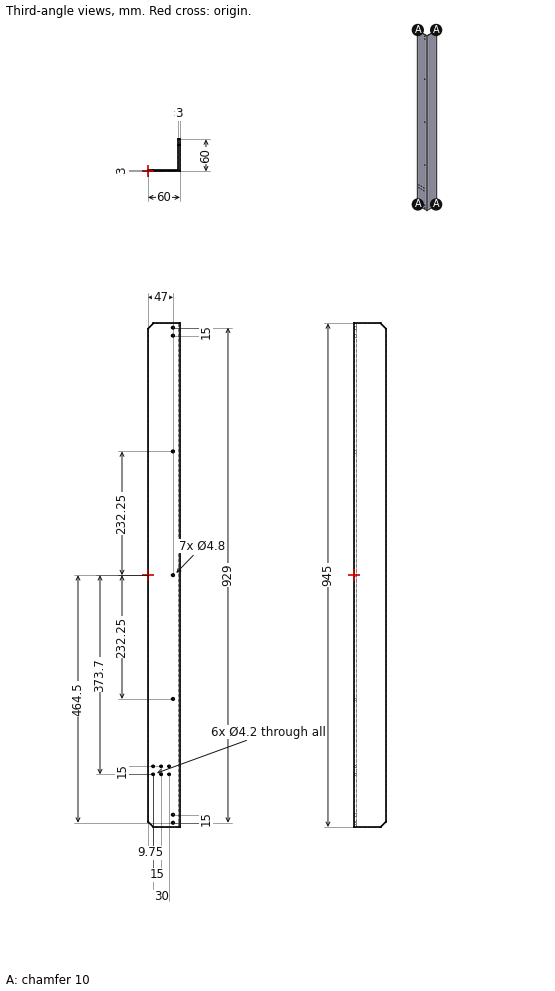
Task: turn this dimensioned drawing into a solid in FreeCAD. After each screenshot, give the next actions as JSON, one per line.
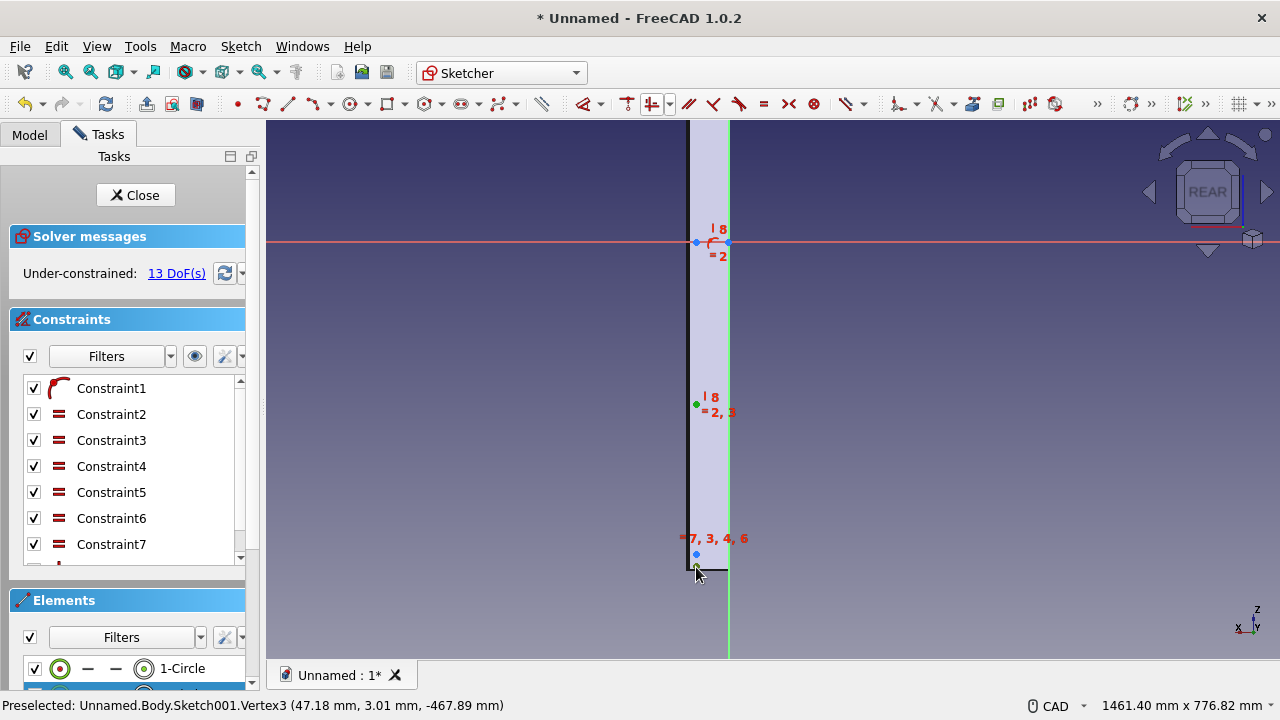
{"action": "key", "text": "v"}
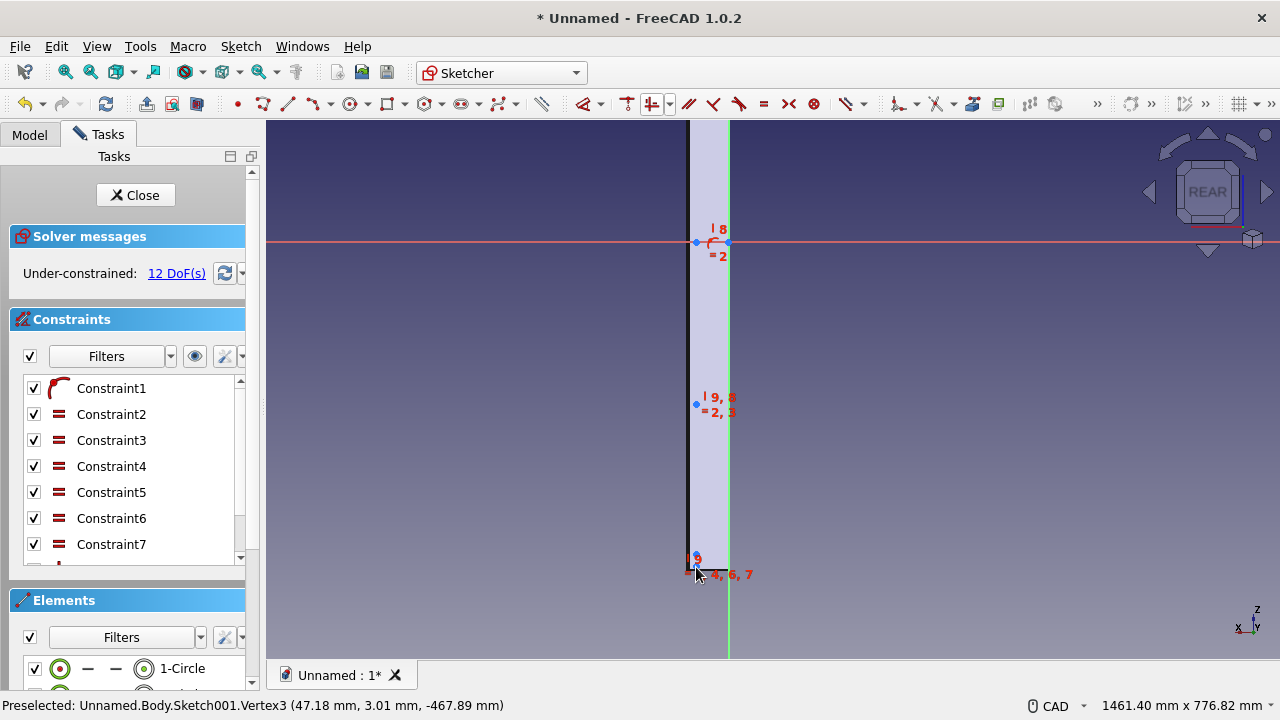
{"action": "left_click", "coordinate": [696, 242]}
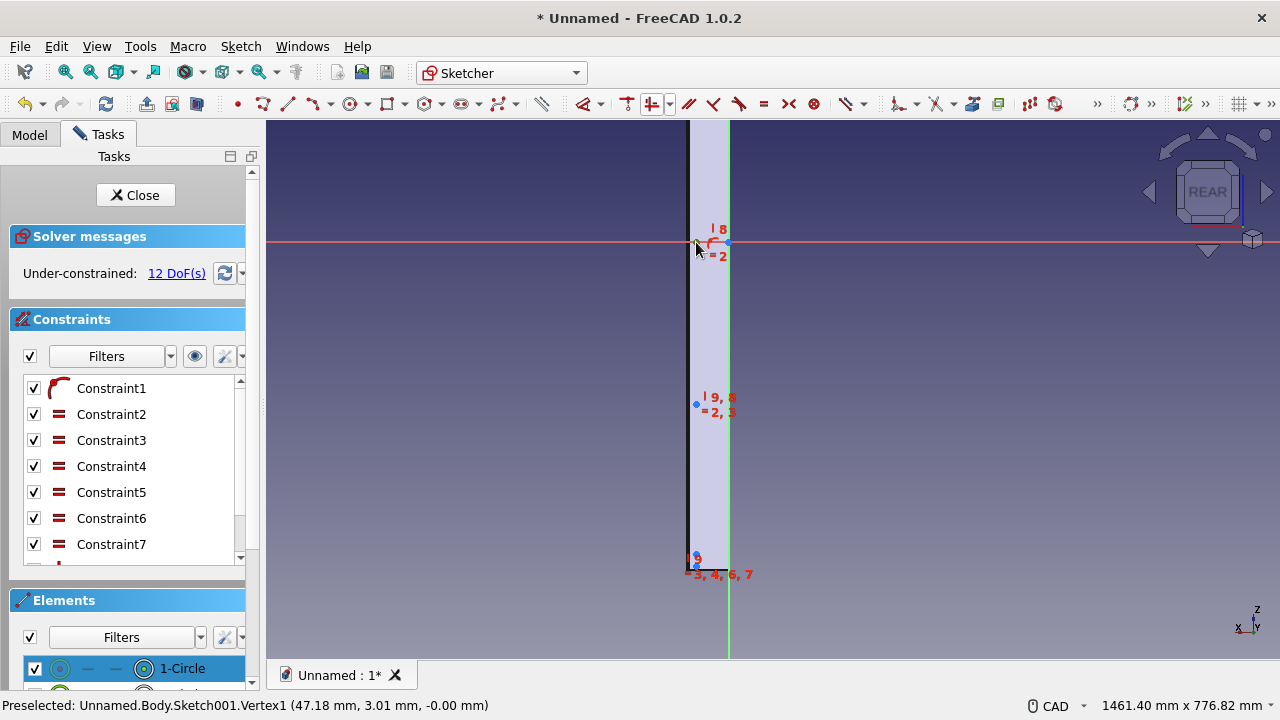
{"action": "scroll", "coordinate": [696, 569], "scroll_direction": "down", "scroll_amount": 3}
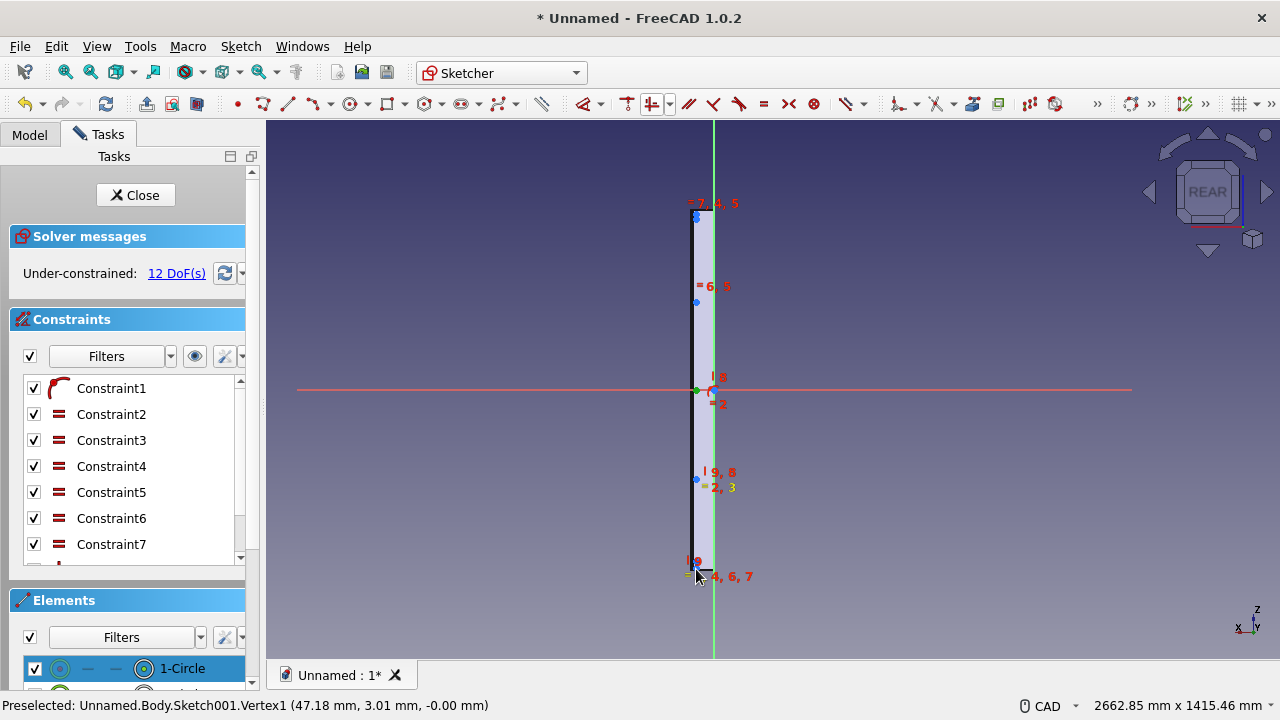
{"action": "scroll", "coordinate": [696, 214], "scroll_direction": "up", "scroll_amount": 5}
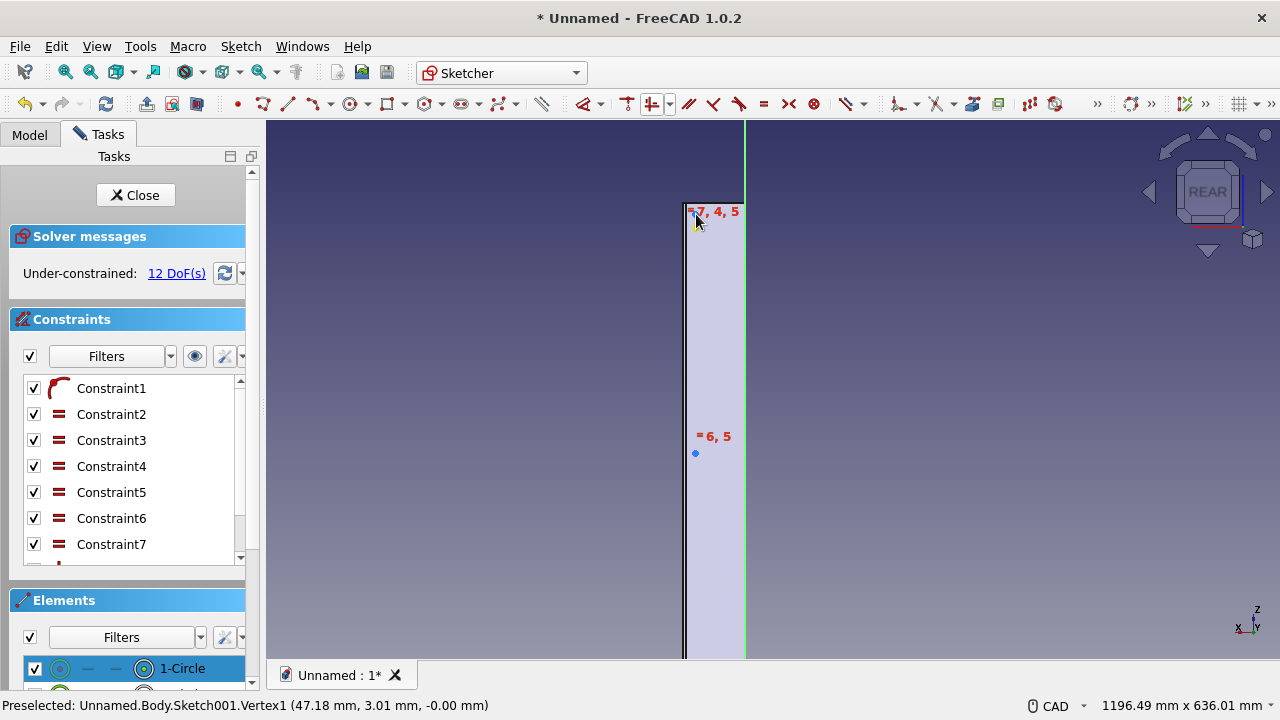
{"action": "scroll", "coordinate": [696, 214], "scroll_direction": "up", "scroll_amount": 4}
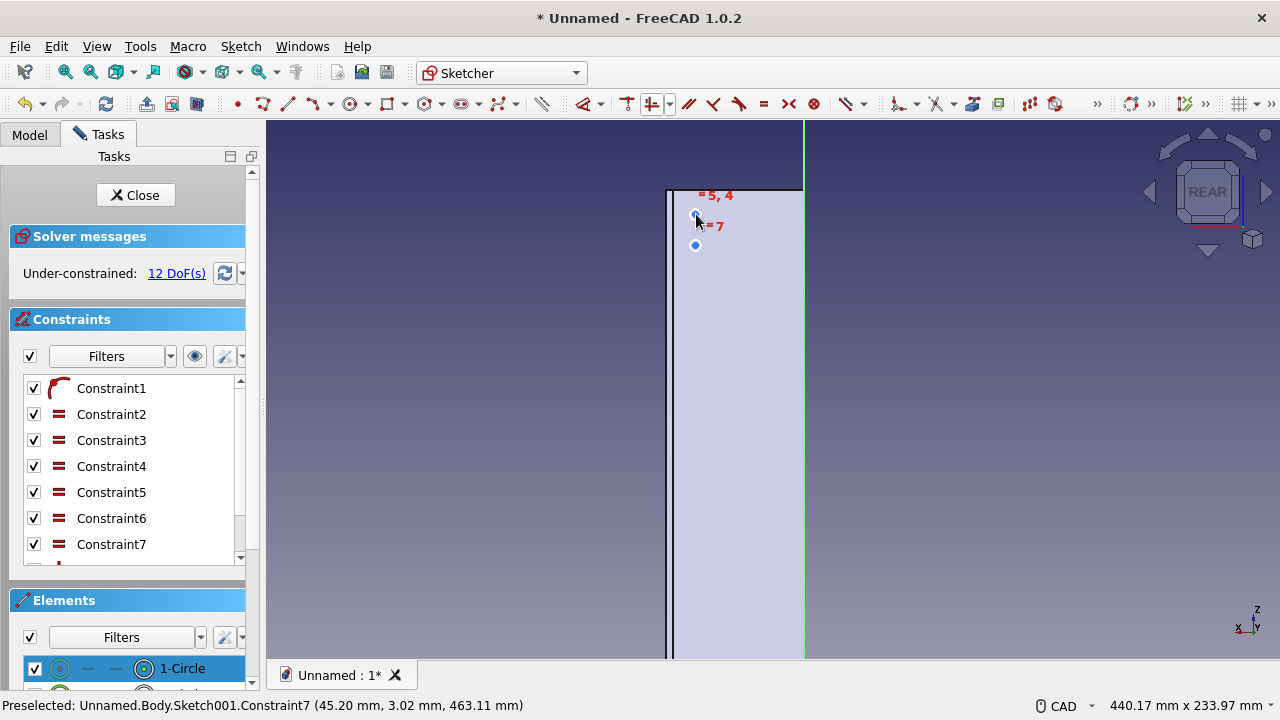
{"action": "left_click", "coordinate": [695, 215]}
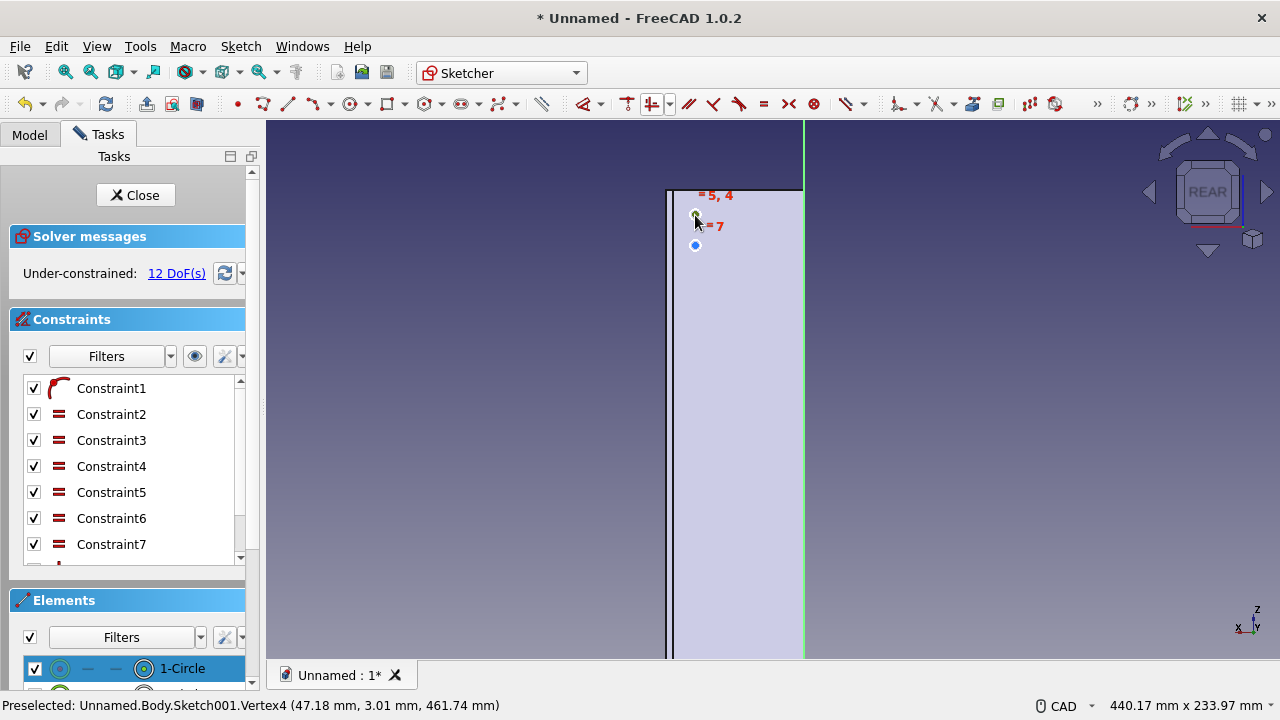
{"action": "left_click", "coordinate": [670, 104]}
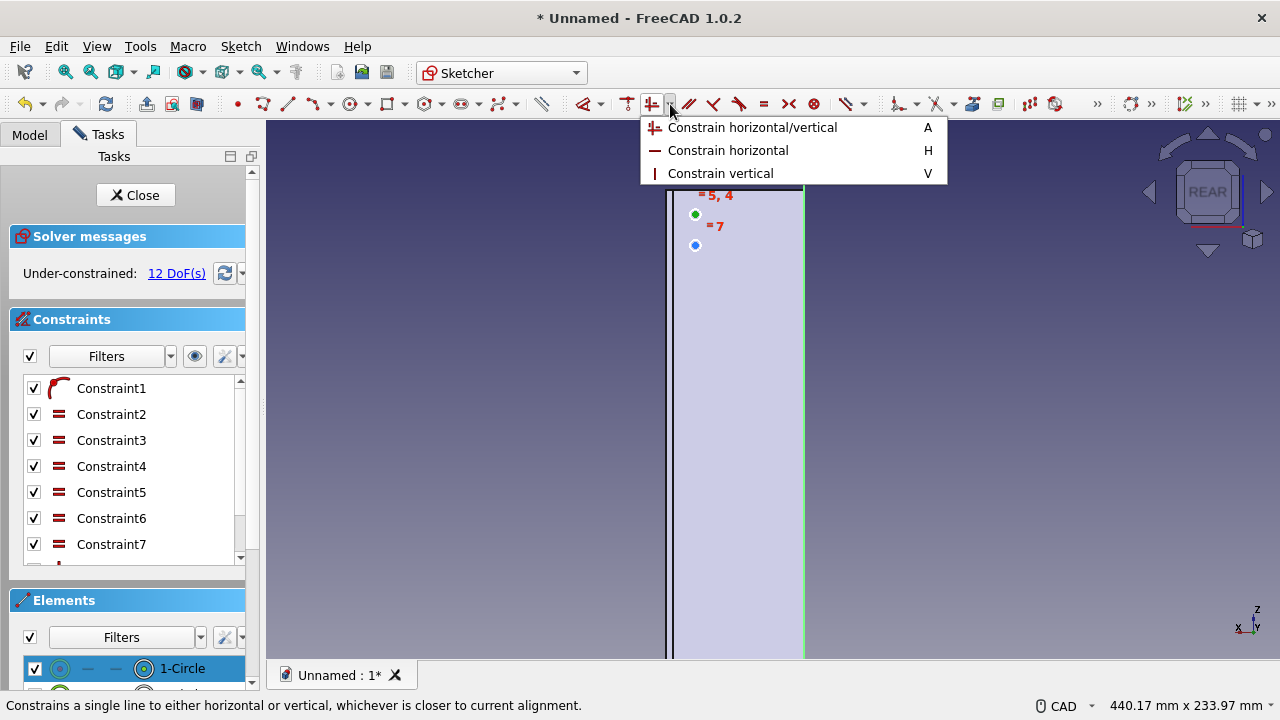
{"action": "left_click", "coordinate": [794, 174]}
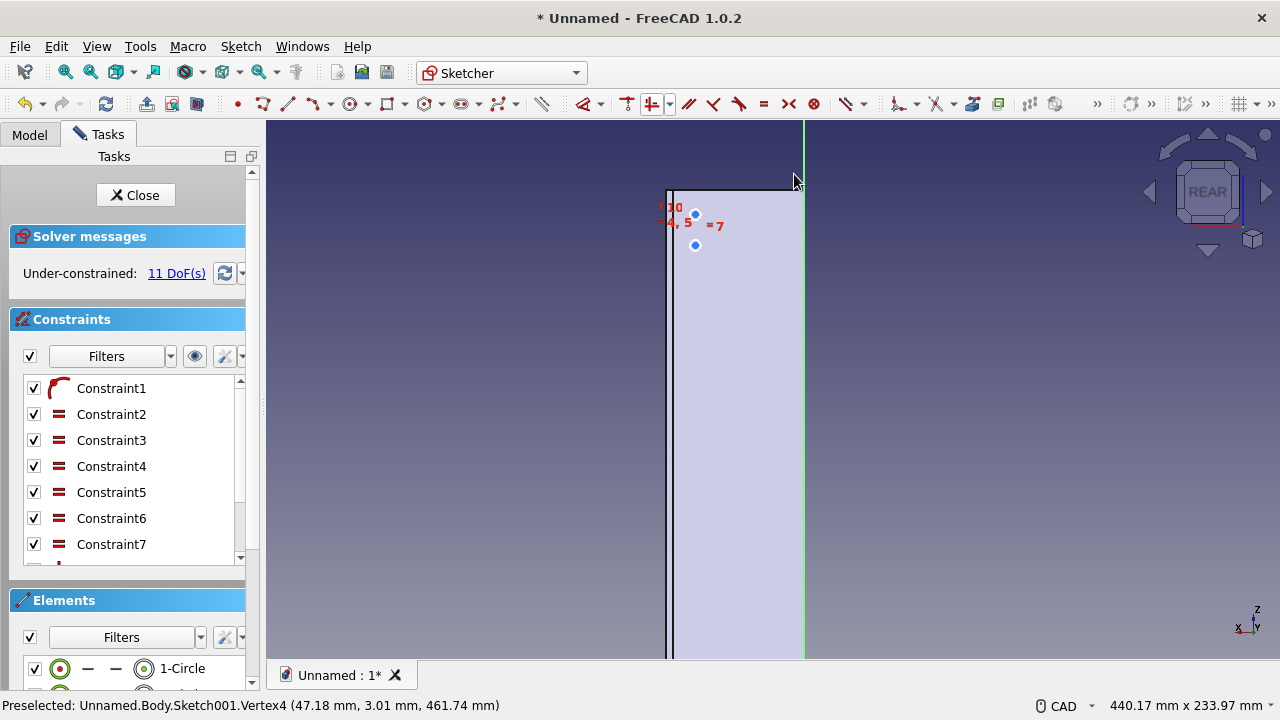
{"action": "scroll", "coordinate": [696, 213], "scroll_direction": "down", "scroll_amount": 9}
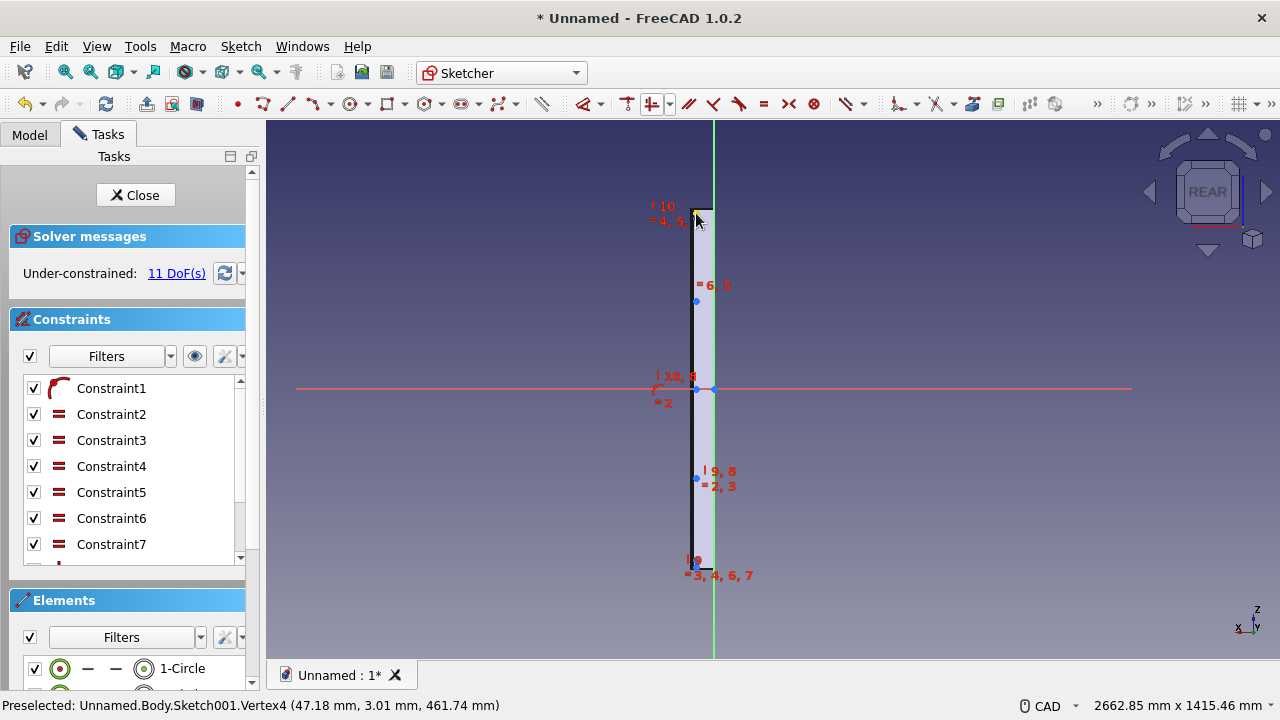
{"action": "left_click", "coordinate": [696, 389]}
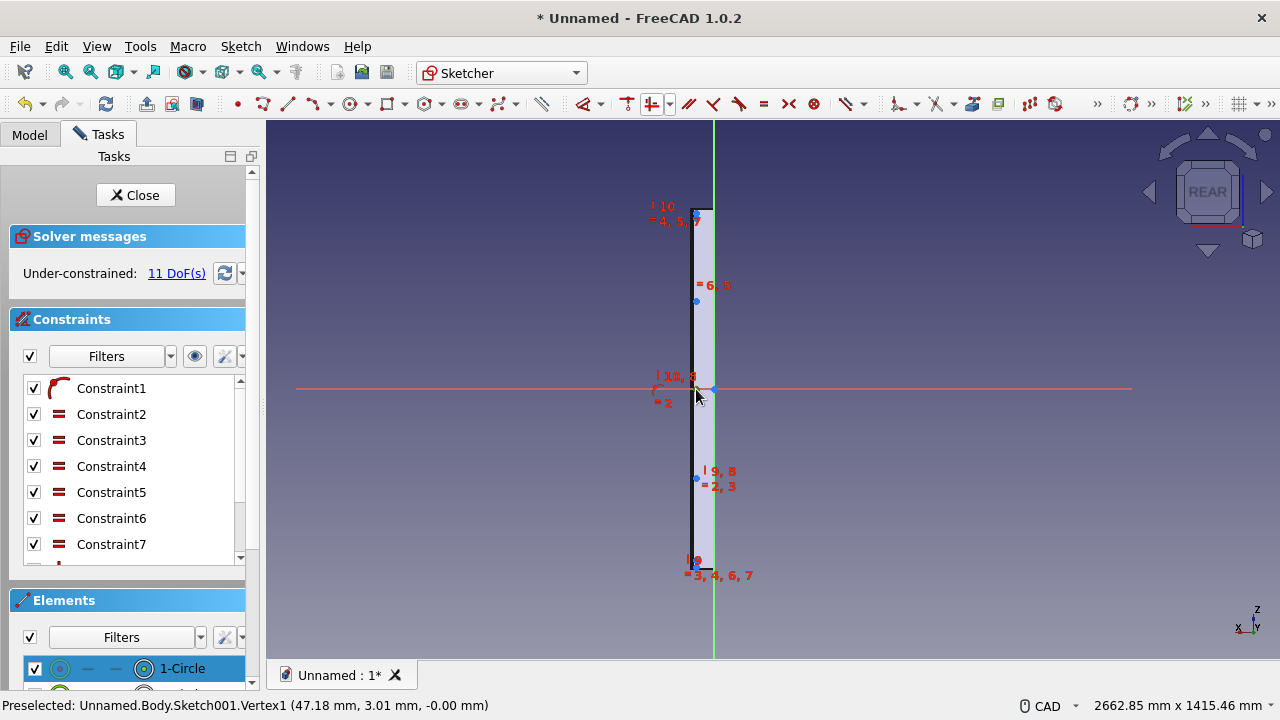
{"action": "left_click", "coordinate": [696, 301]}